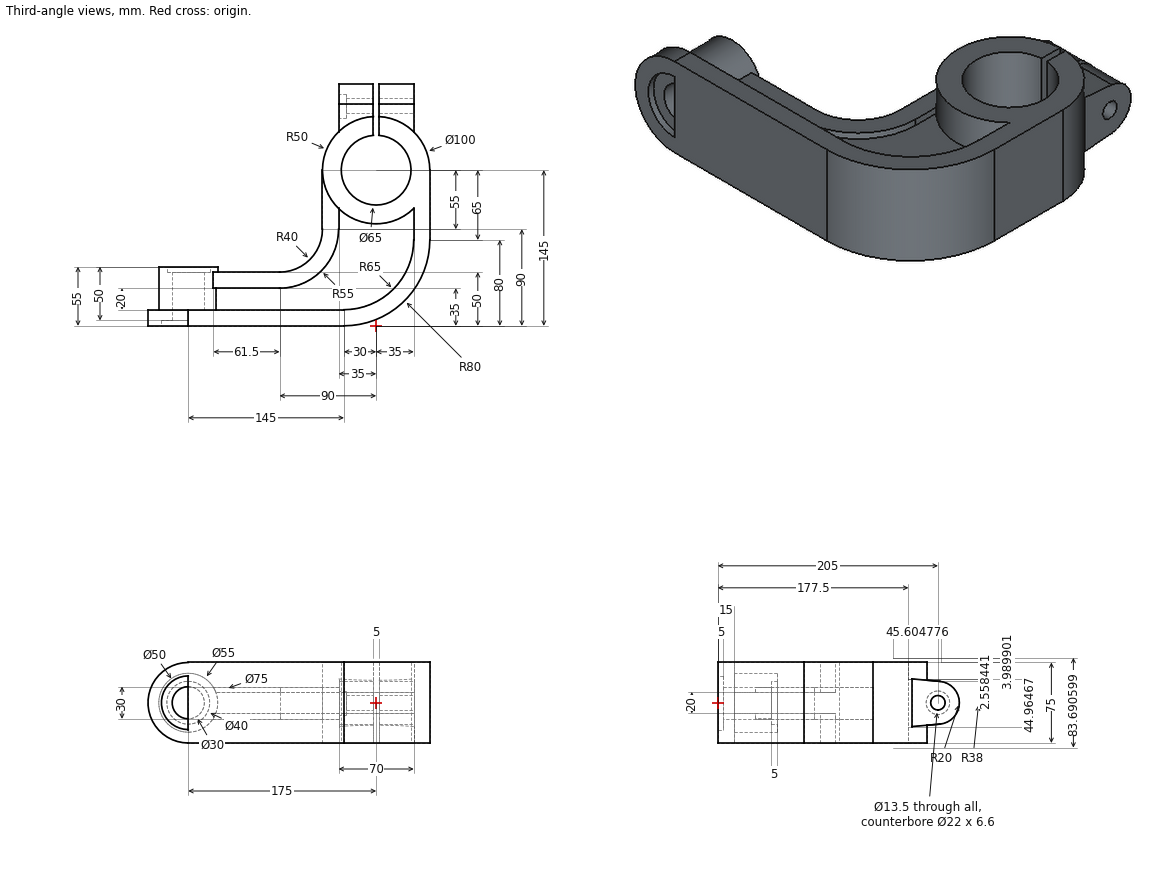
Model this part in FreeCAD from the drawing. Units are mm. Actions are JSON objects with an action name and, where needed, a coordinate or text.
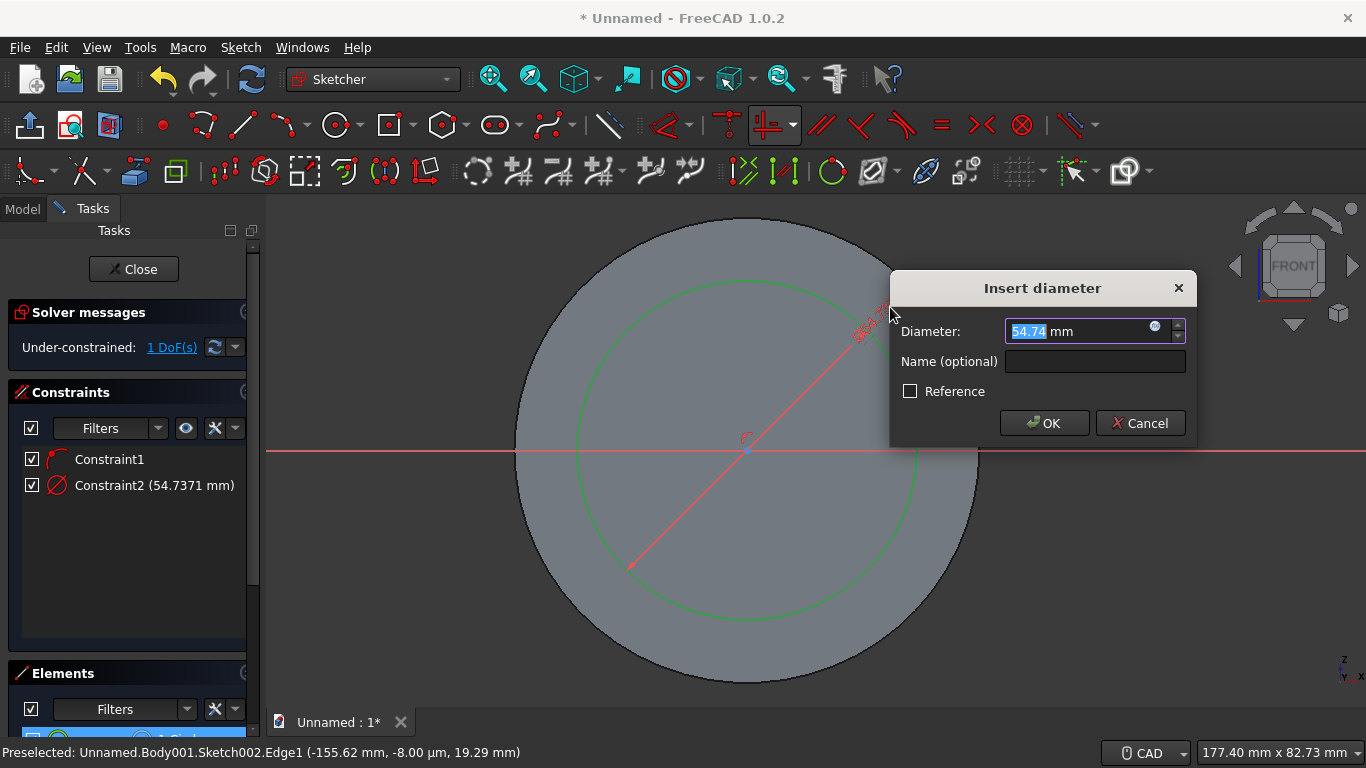
{"action": "type", "text": "55"}
{"action": "key", "text": "Return"}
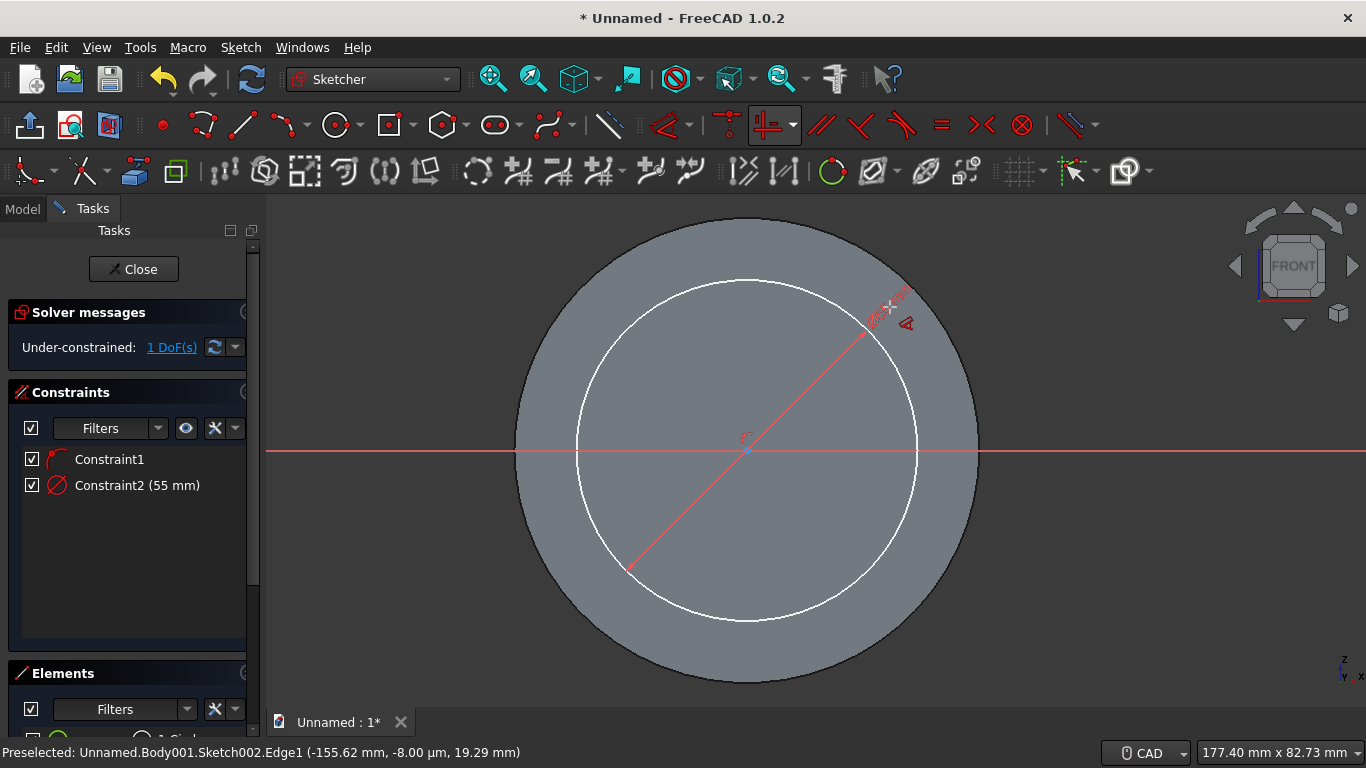
{"action": "left_click", "coordinate": [747, 450]}
{"action": "left_click", "coordinate": [974, 484]}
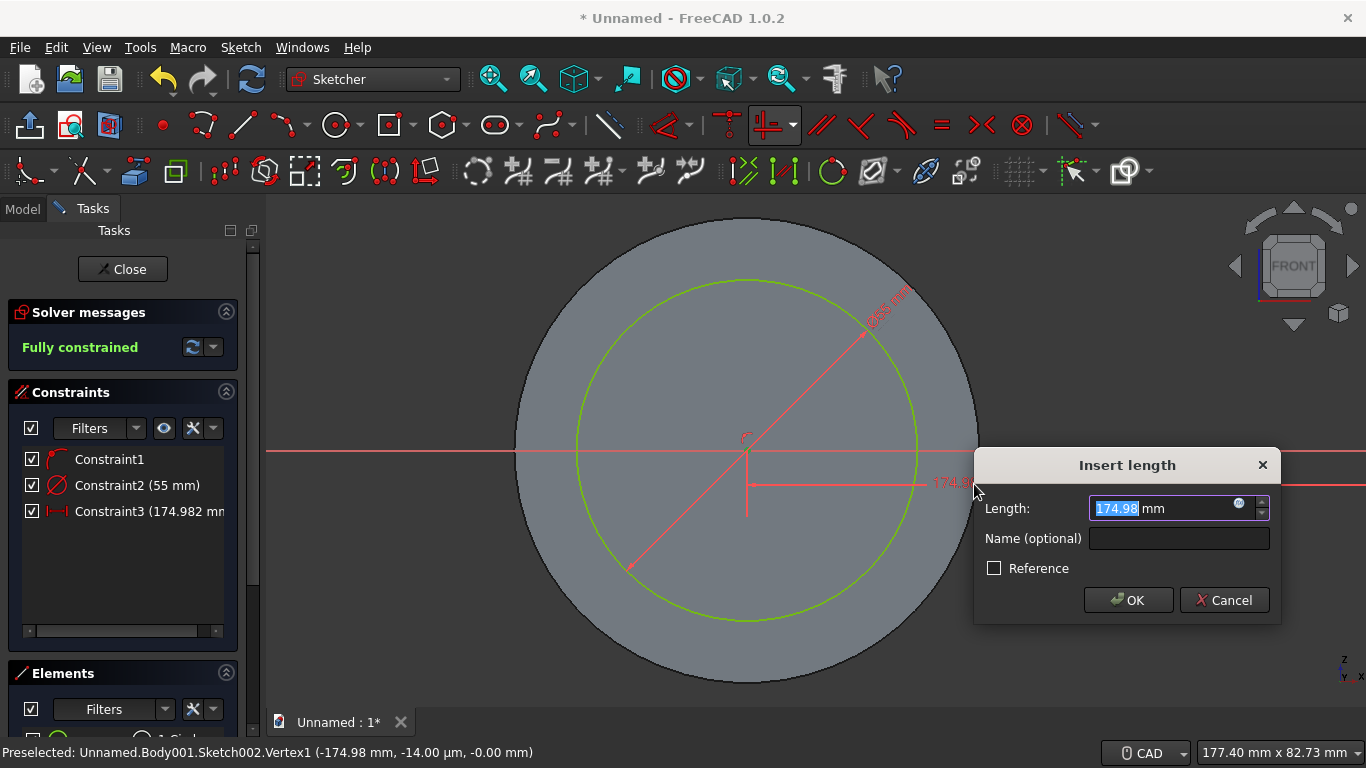
{"action": "type", "text": "175"}
{"action": "key", "text": "Return"}
{"action": "key", "text": "Escape"}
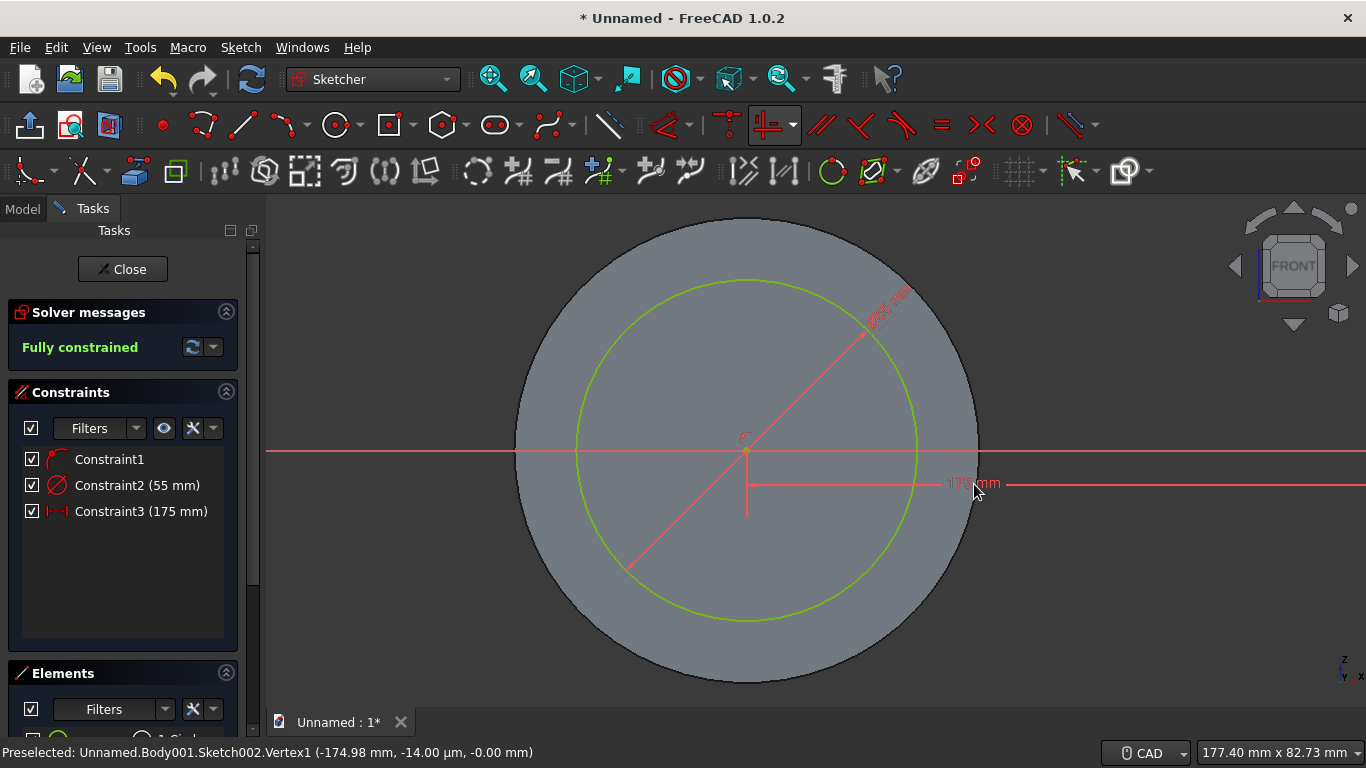
{"action": "left_click", "coordinate": [123, 269]}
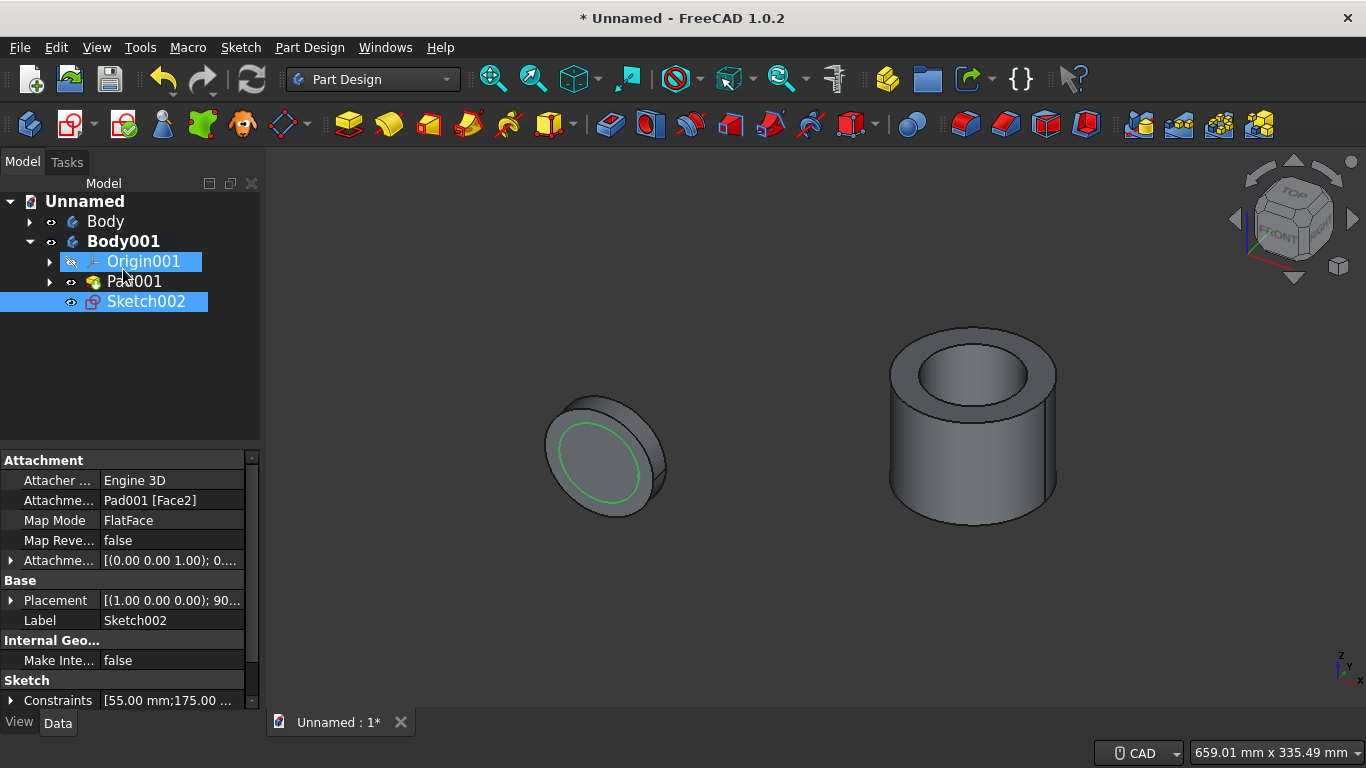
{"action": "left_click", "coordinate": [350, 124]}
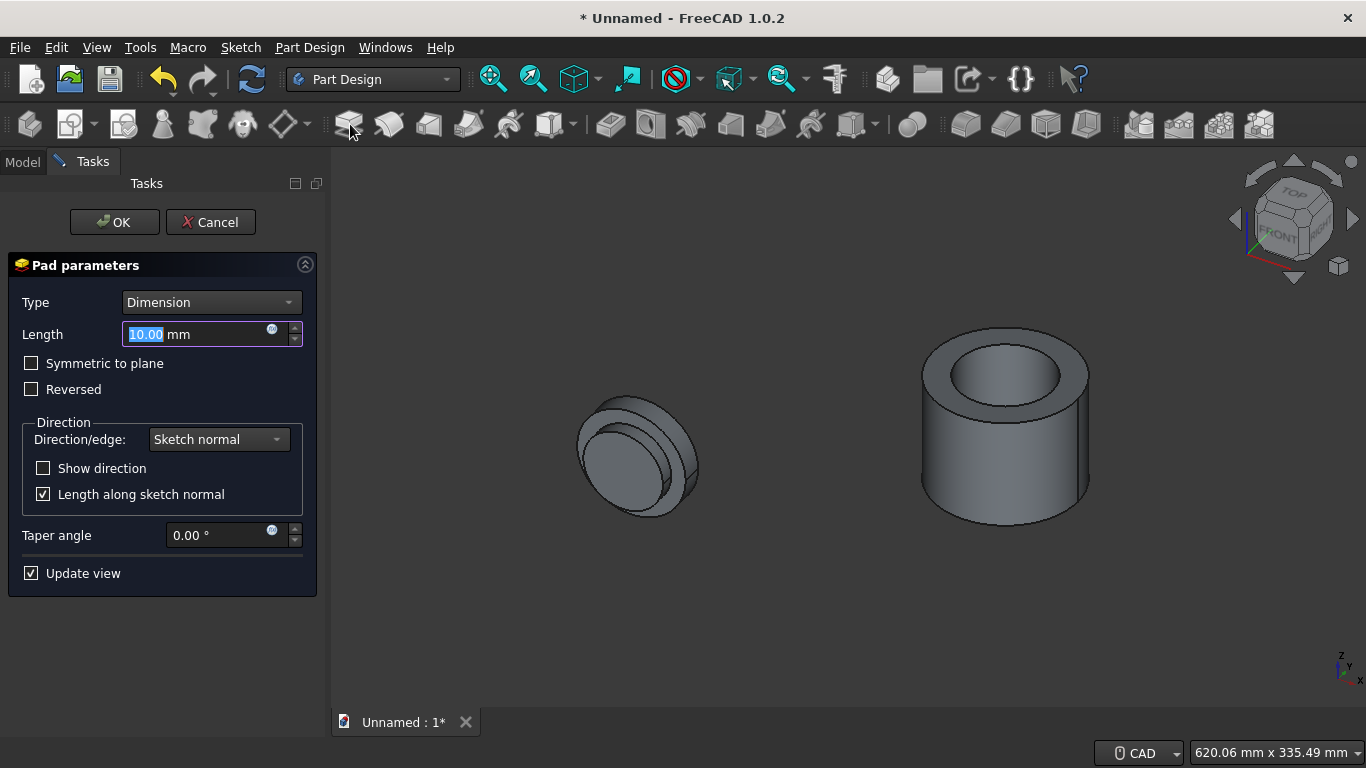
{"action": "type", "text": "55"}
{"action": "key", "text": "Tab"}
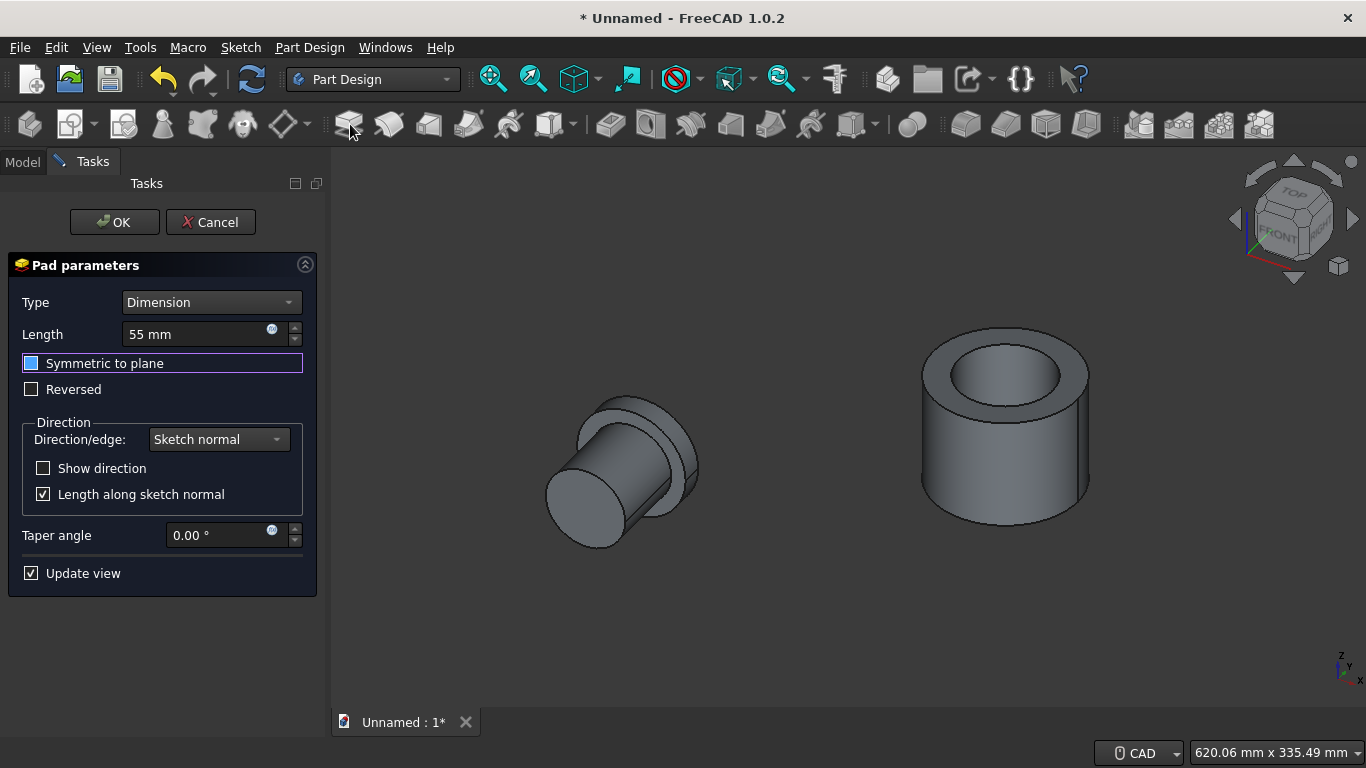
{"action": "left_click", "coordinate": [30, 389]}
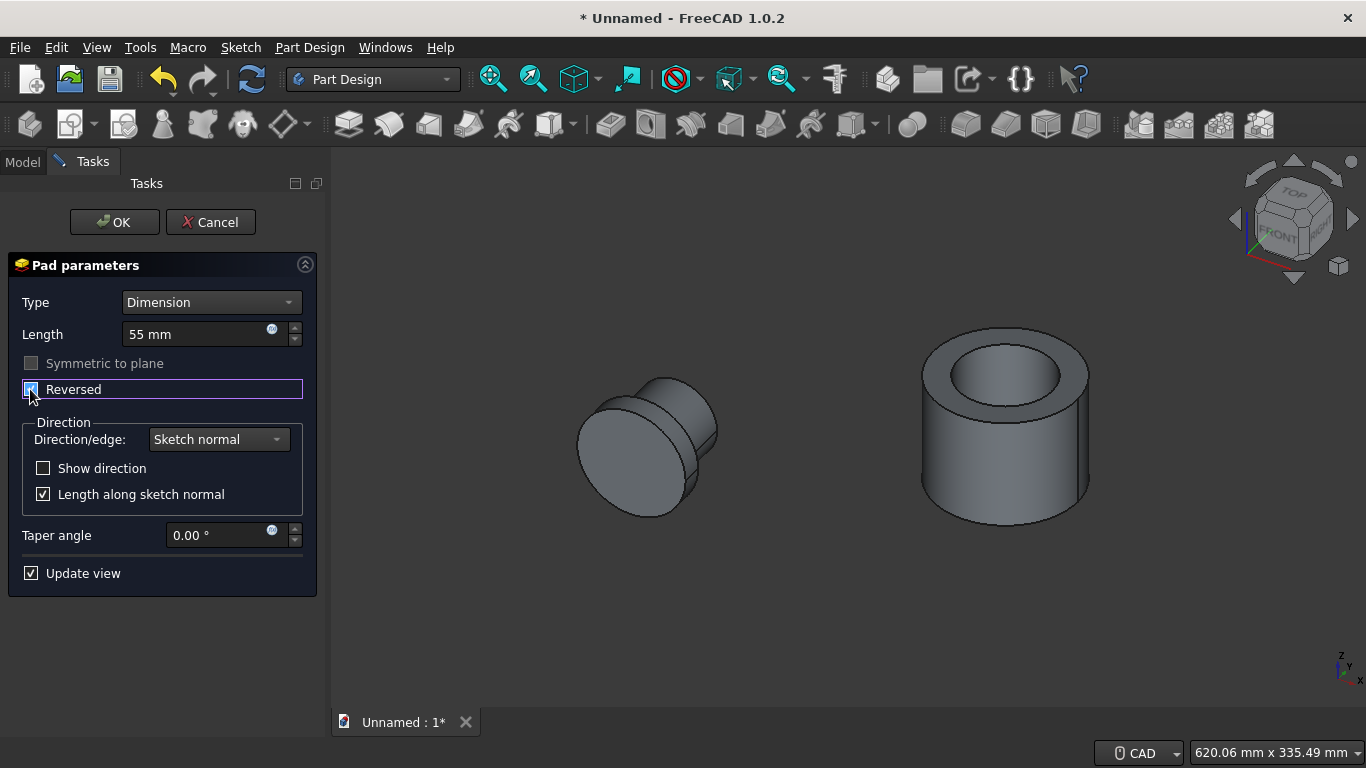
{"action": "left_click", "coordinate": [115, 222]}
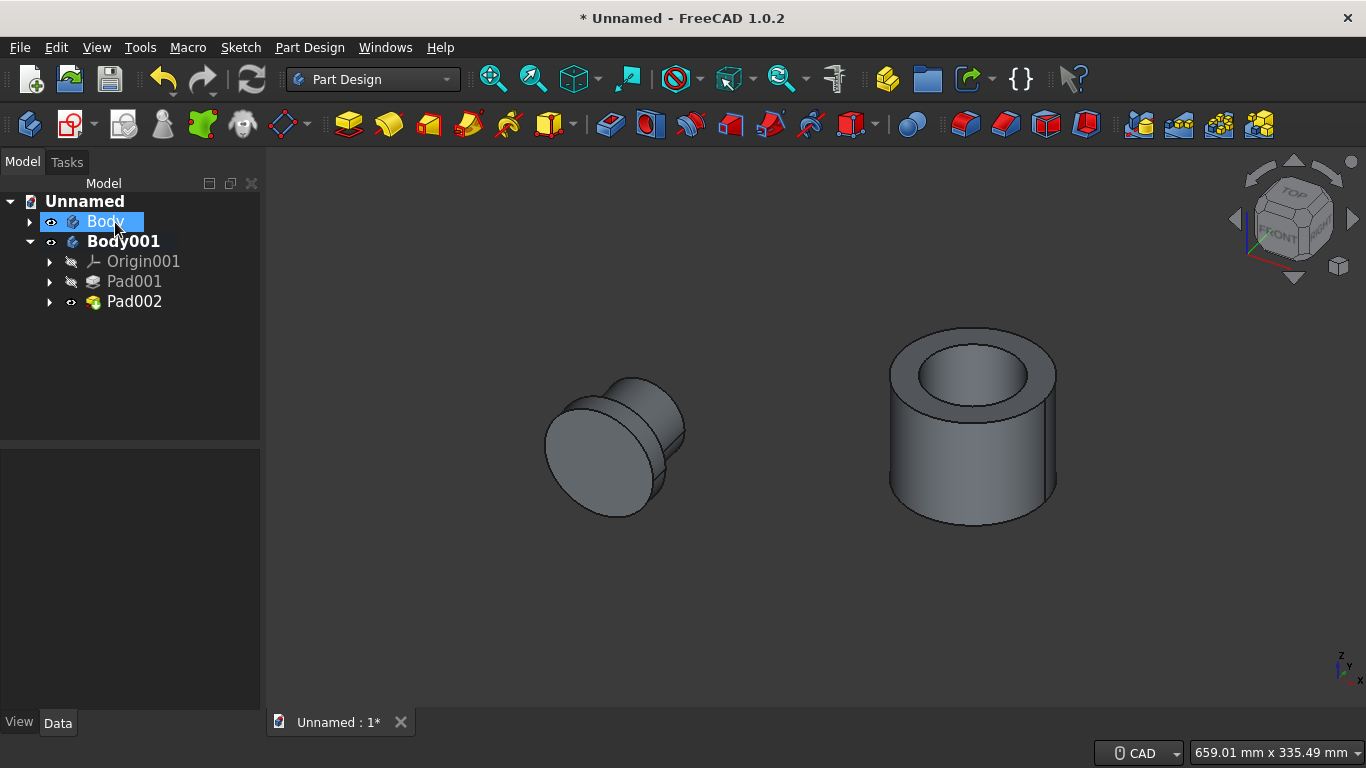
{"action": "key", "text": "v f"}